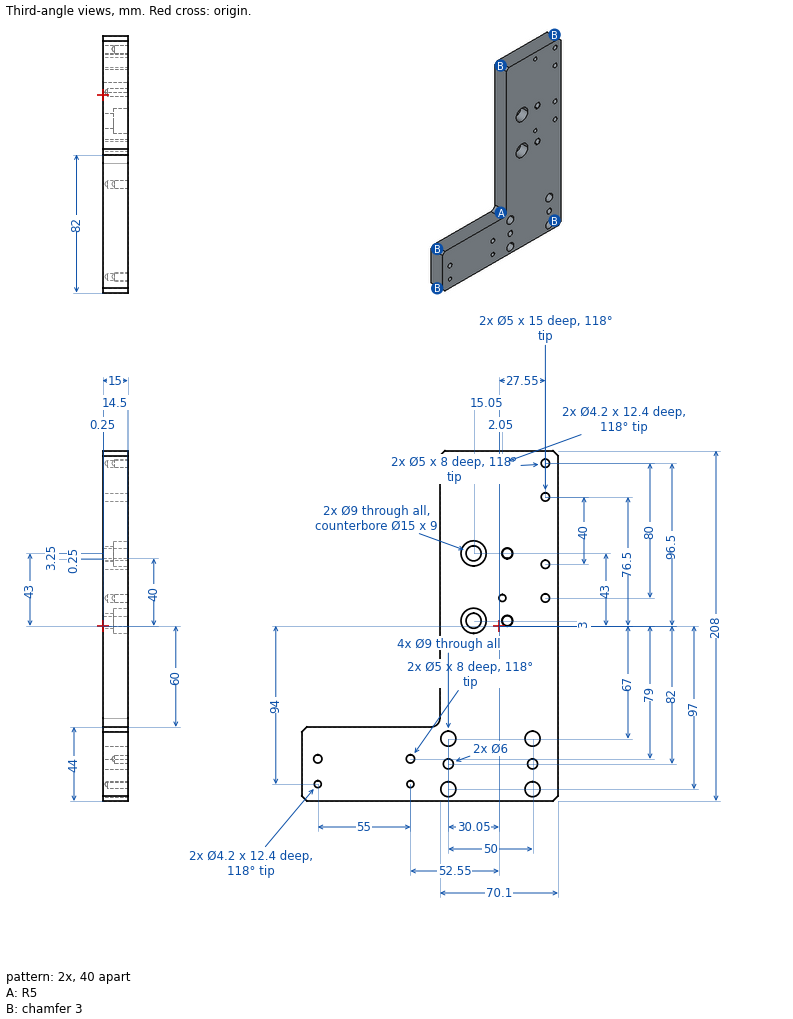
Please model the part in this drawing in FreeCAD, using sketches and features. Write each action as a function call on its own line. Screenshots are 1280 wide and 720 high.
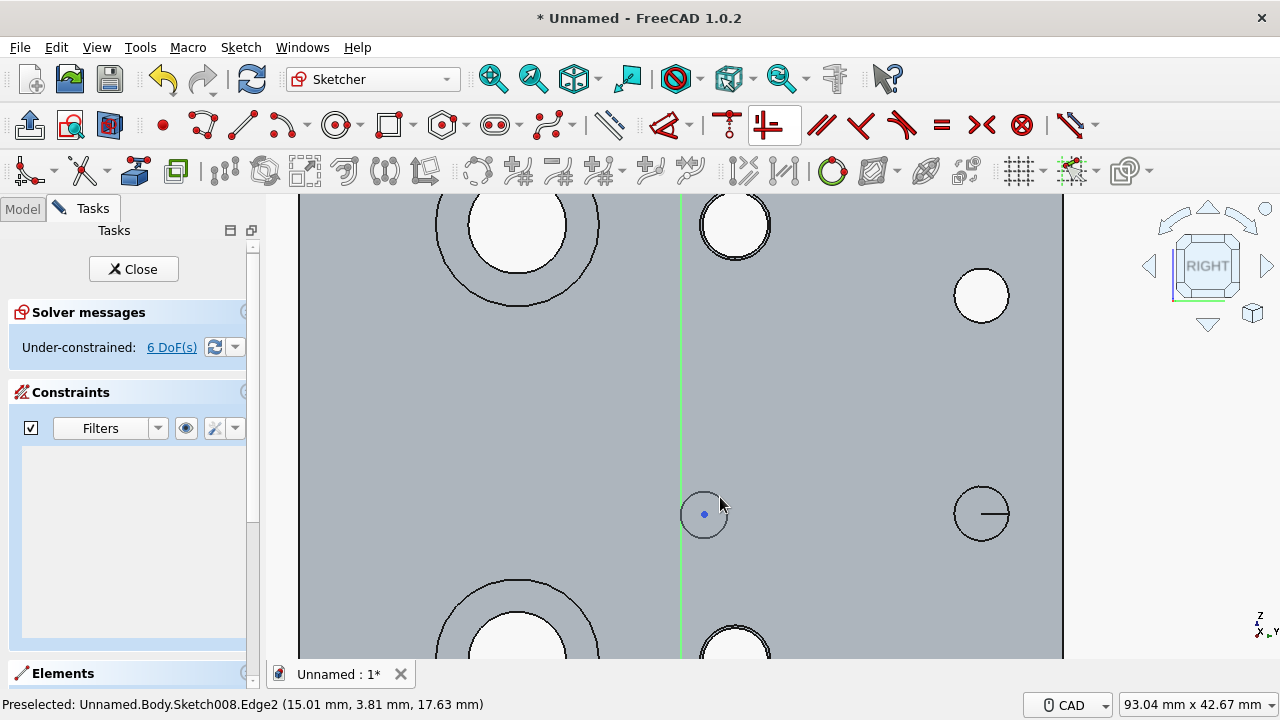
scroll(705, 515, down, 7)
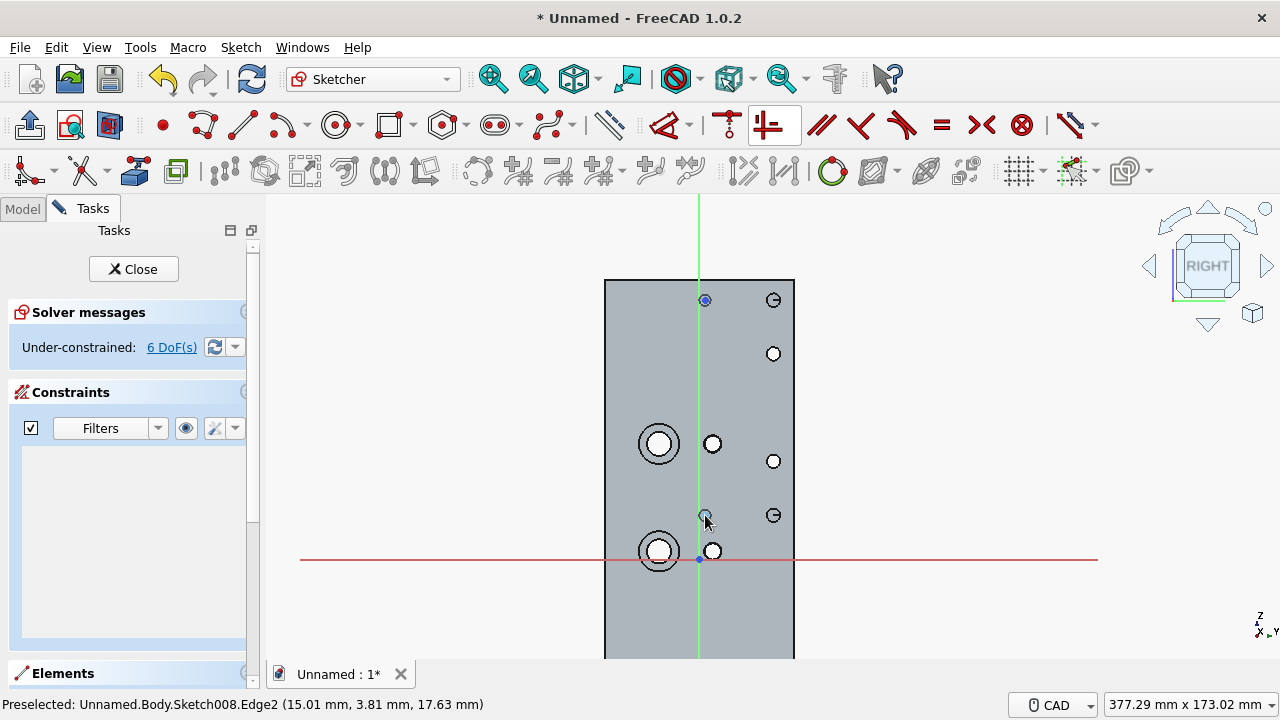
scroll(709, 296, up, 5)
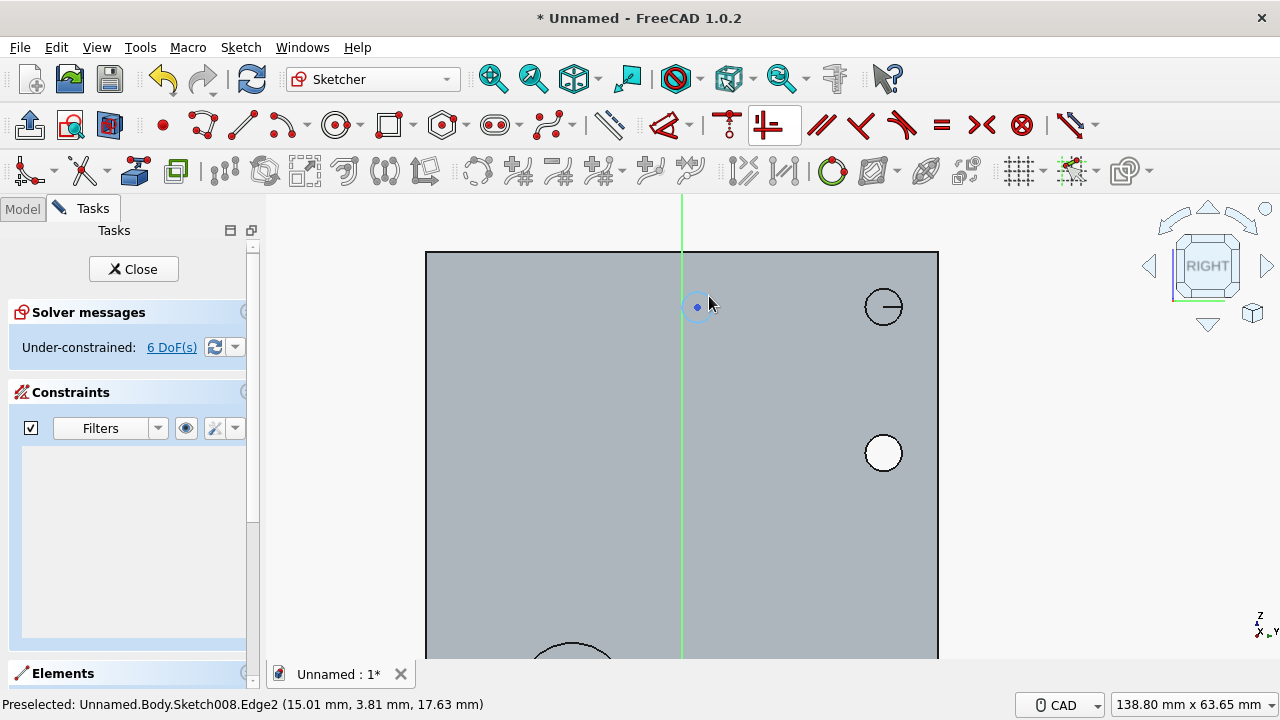
click(708, 297)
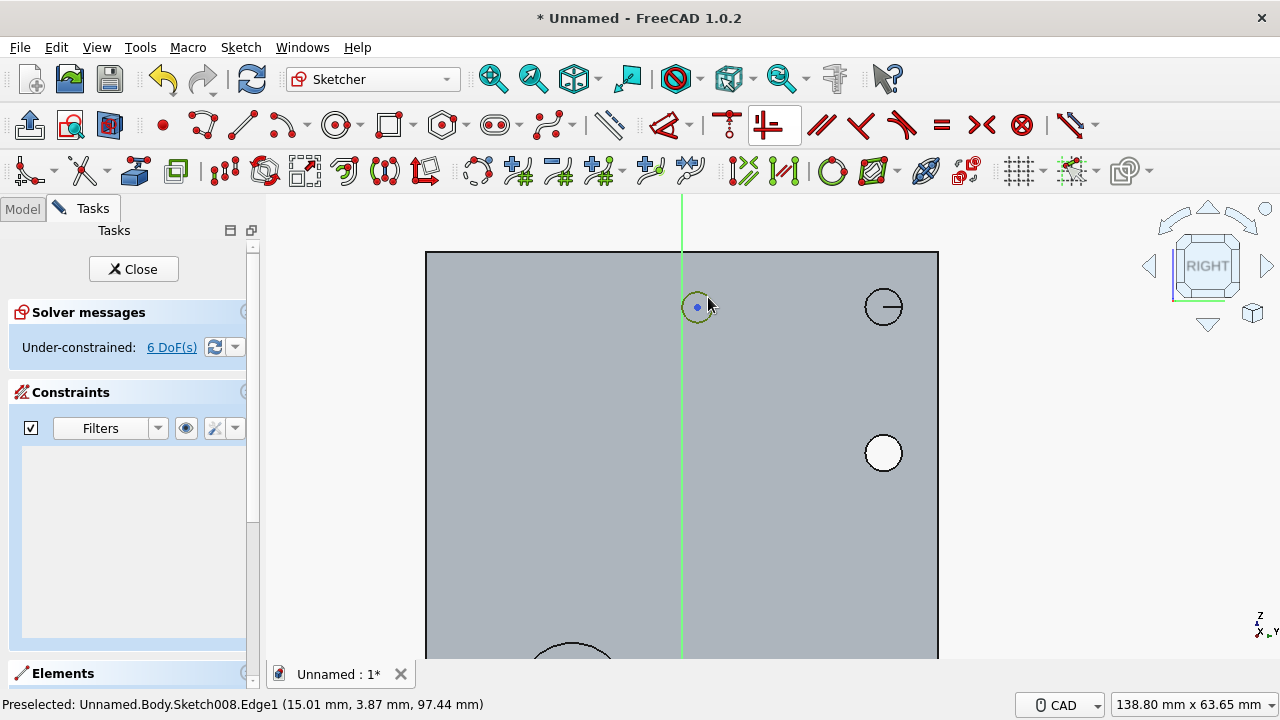
scroll(709, 295, down, 5)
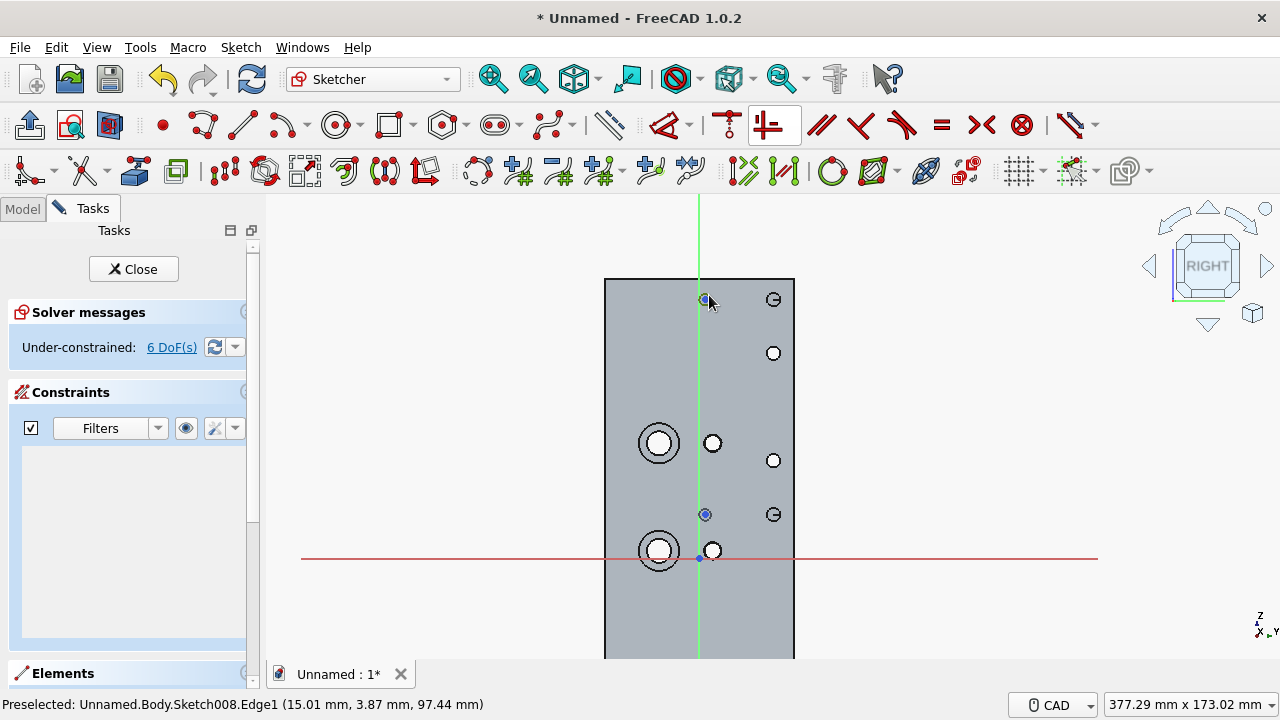
scroll(709, 511, up, 5)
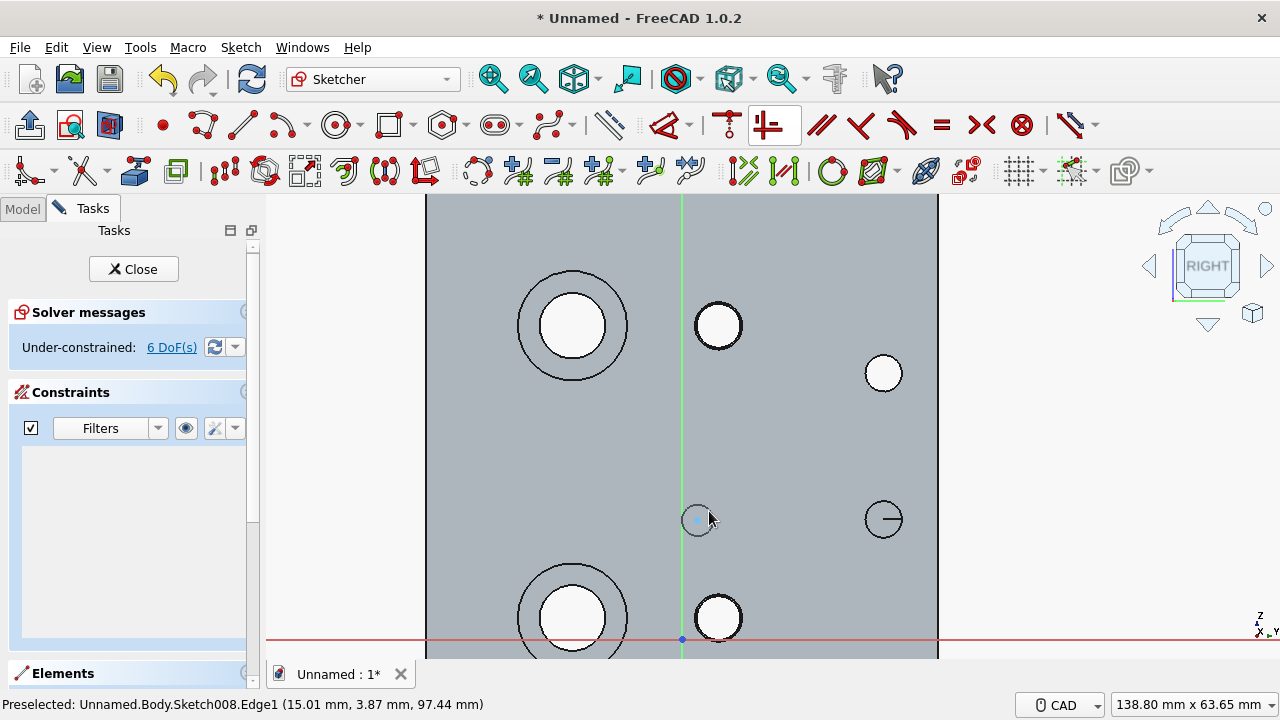
click(709, 509)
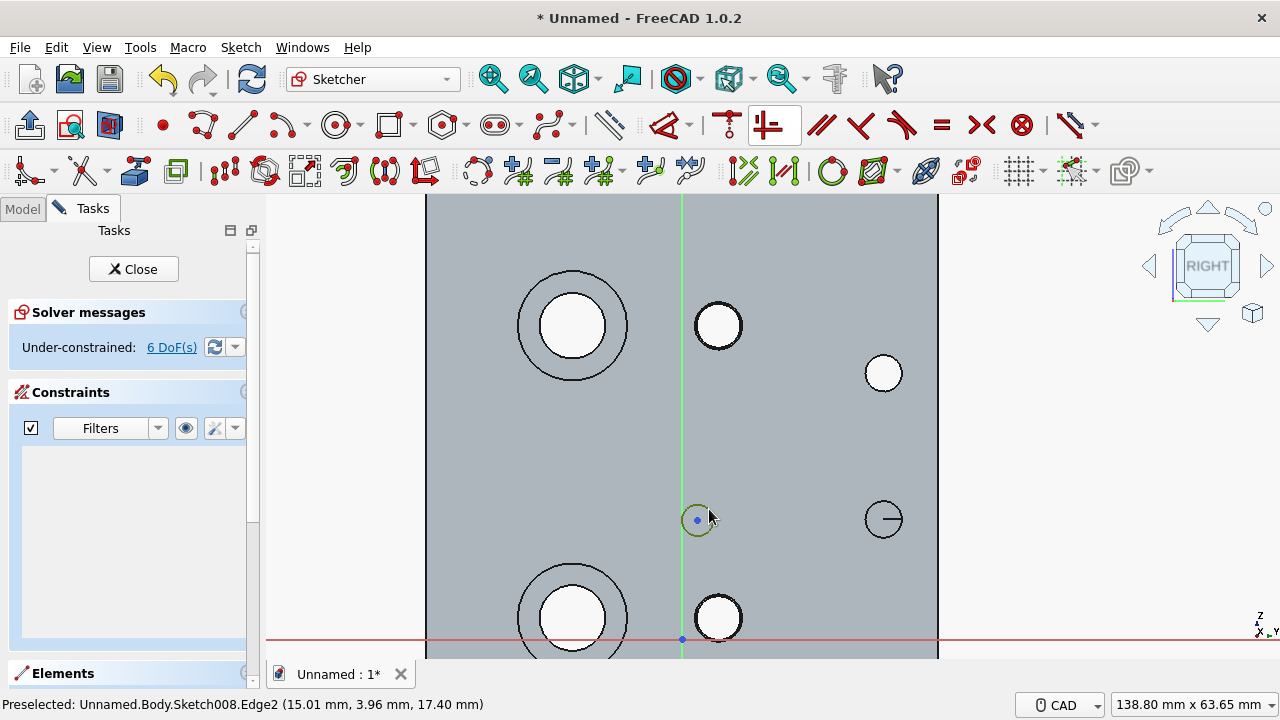
click(942, 126)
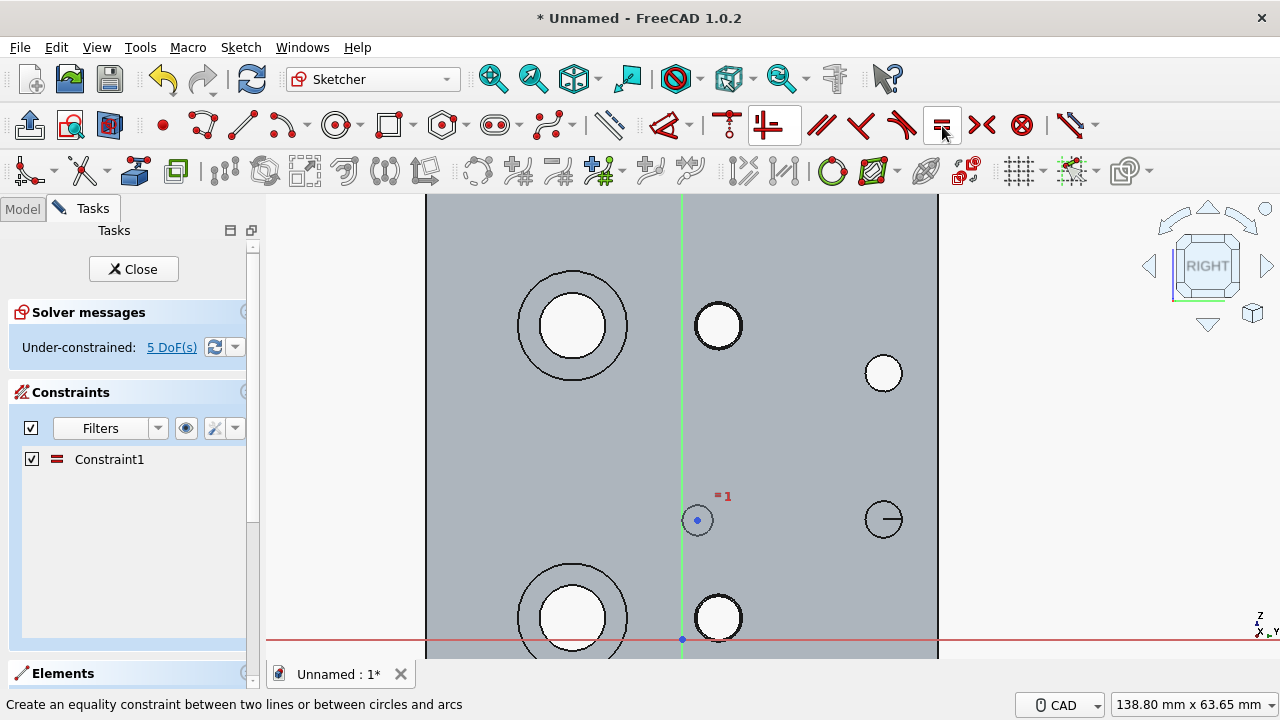
scroll(709, 512, down, 5)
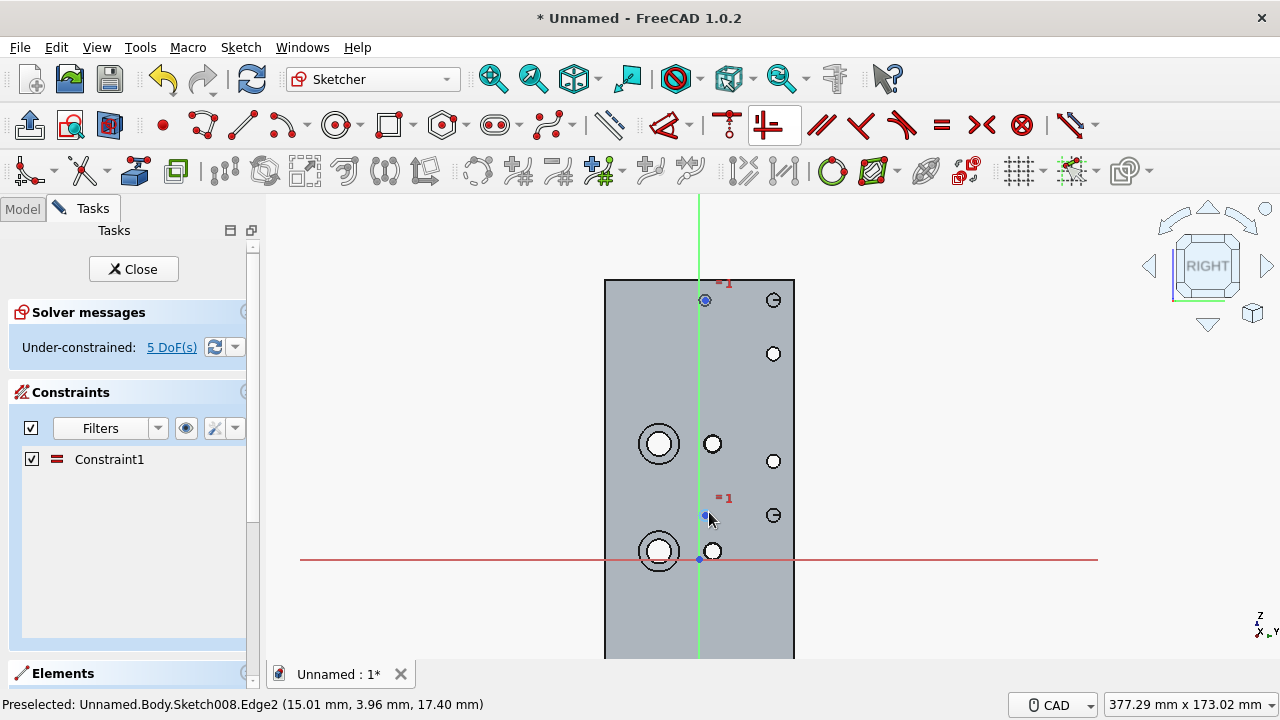
click(705, 300)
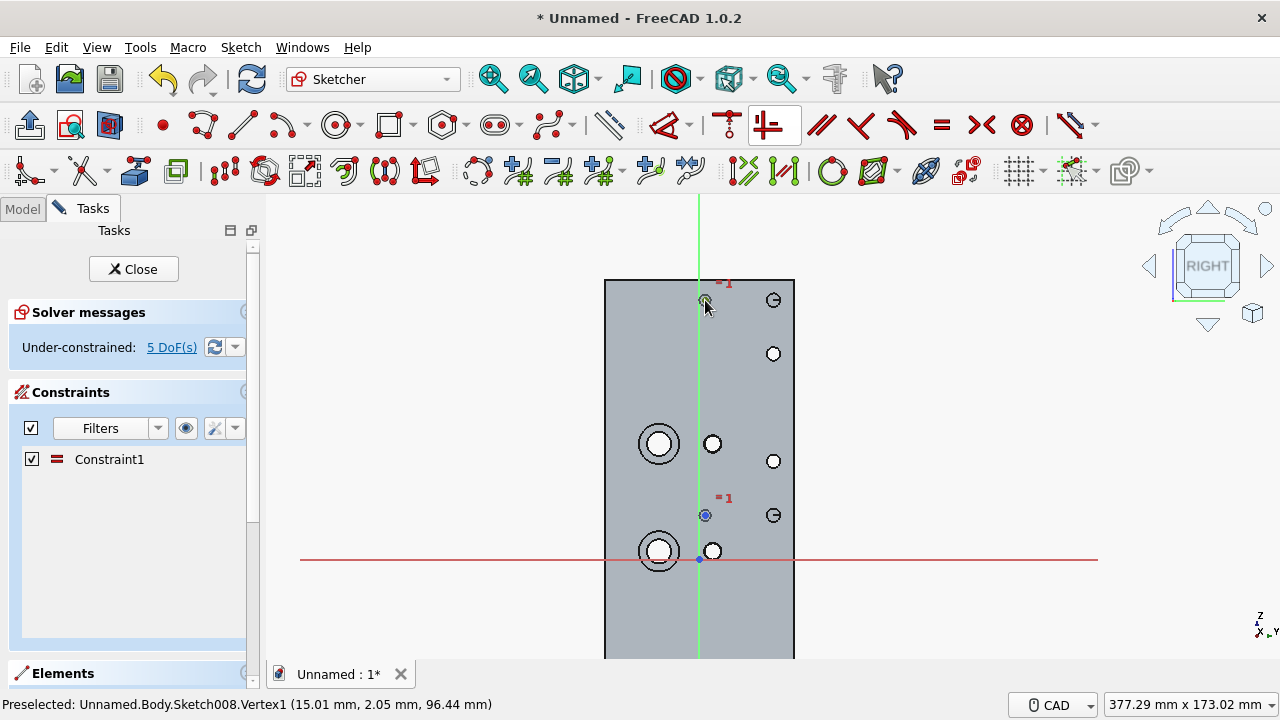
click(705, 516)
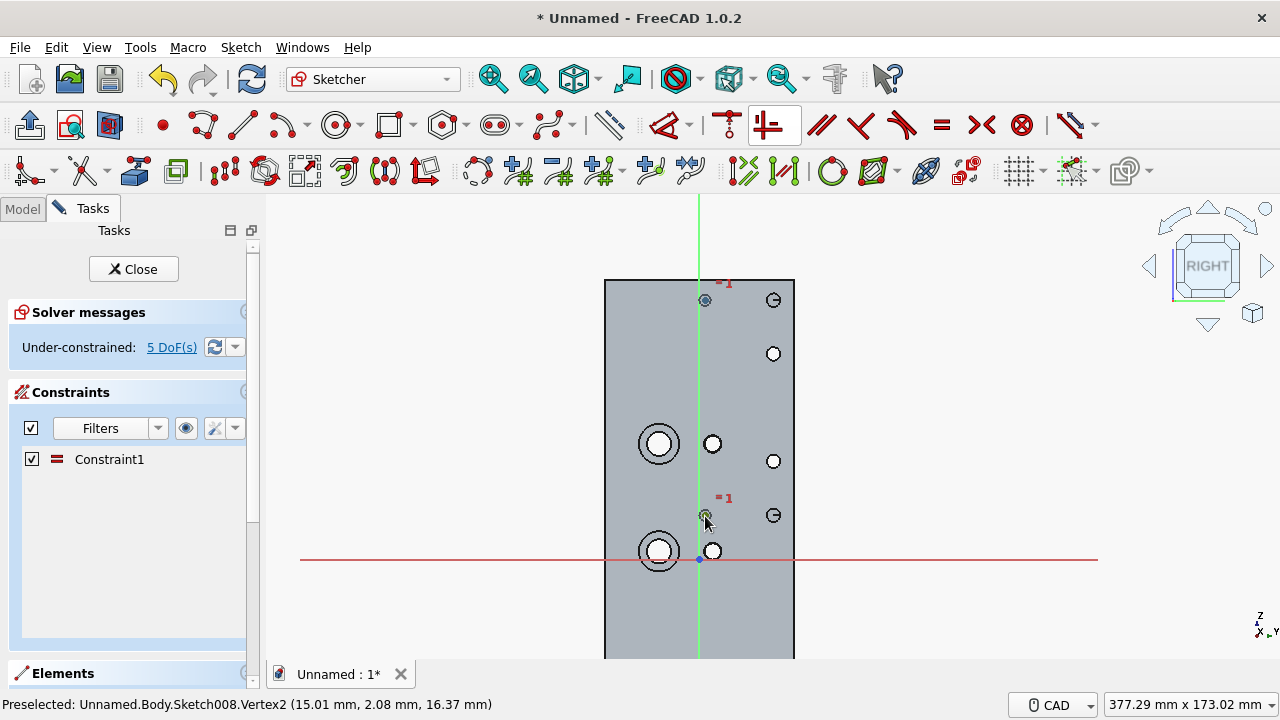
click(796, 126)